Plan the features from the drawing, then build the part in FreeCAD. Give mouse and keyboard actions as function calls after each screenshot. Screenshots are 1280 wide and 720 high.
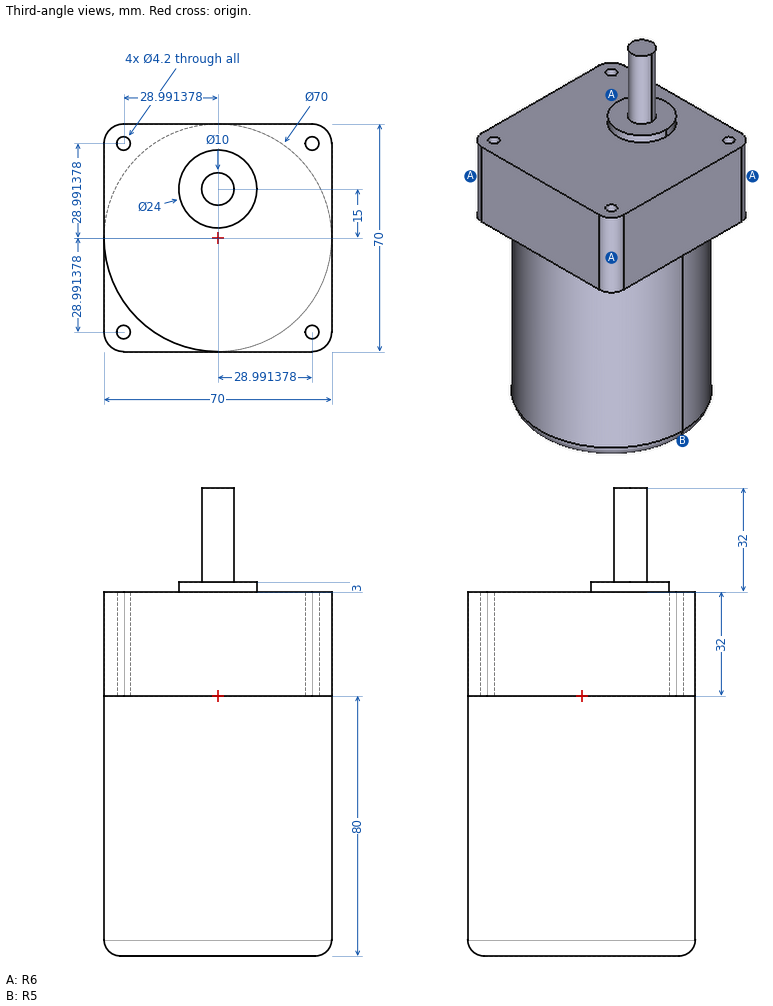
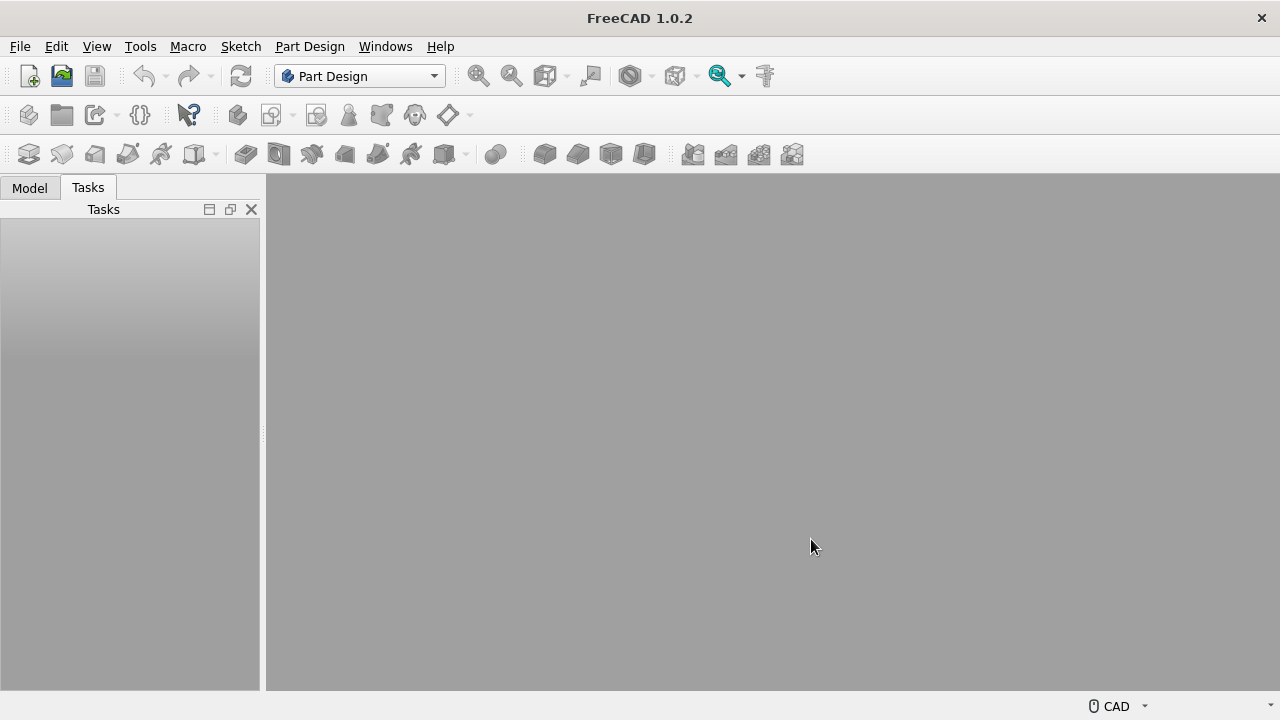
click(29, 76)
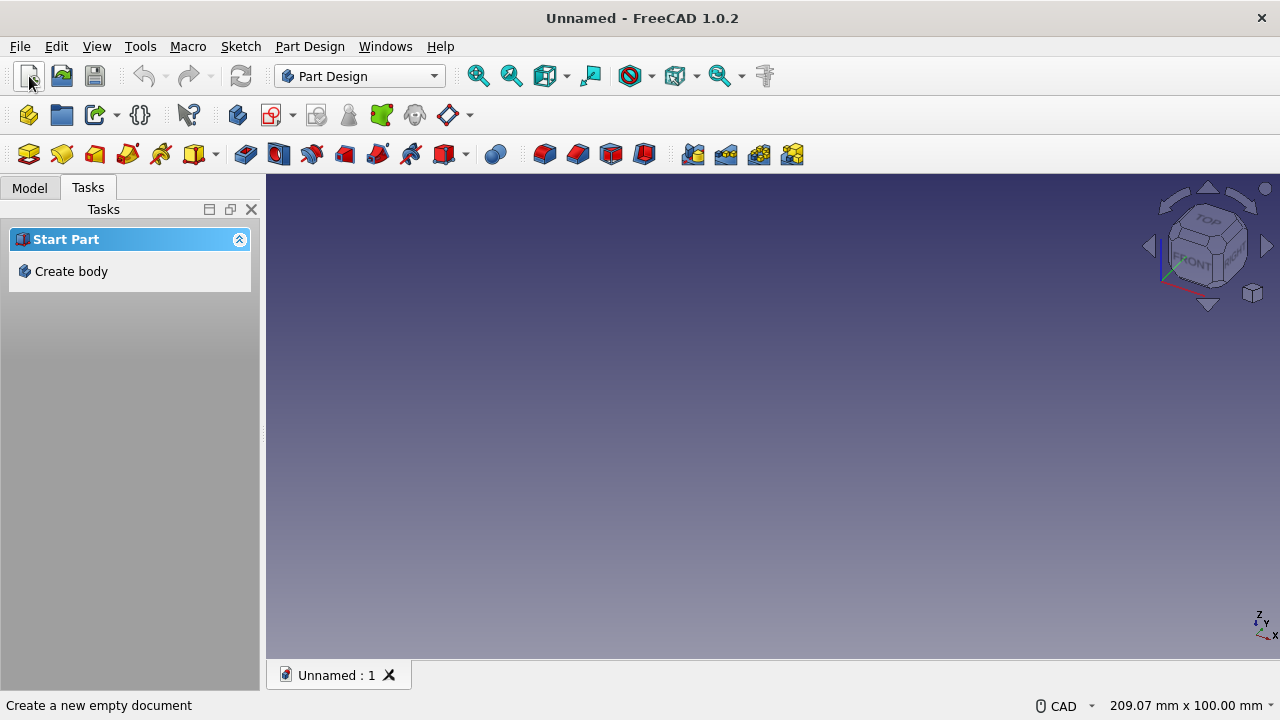
click(270, 116)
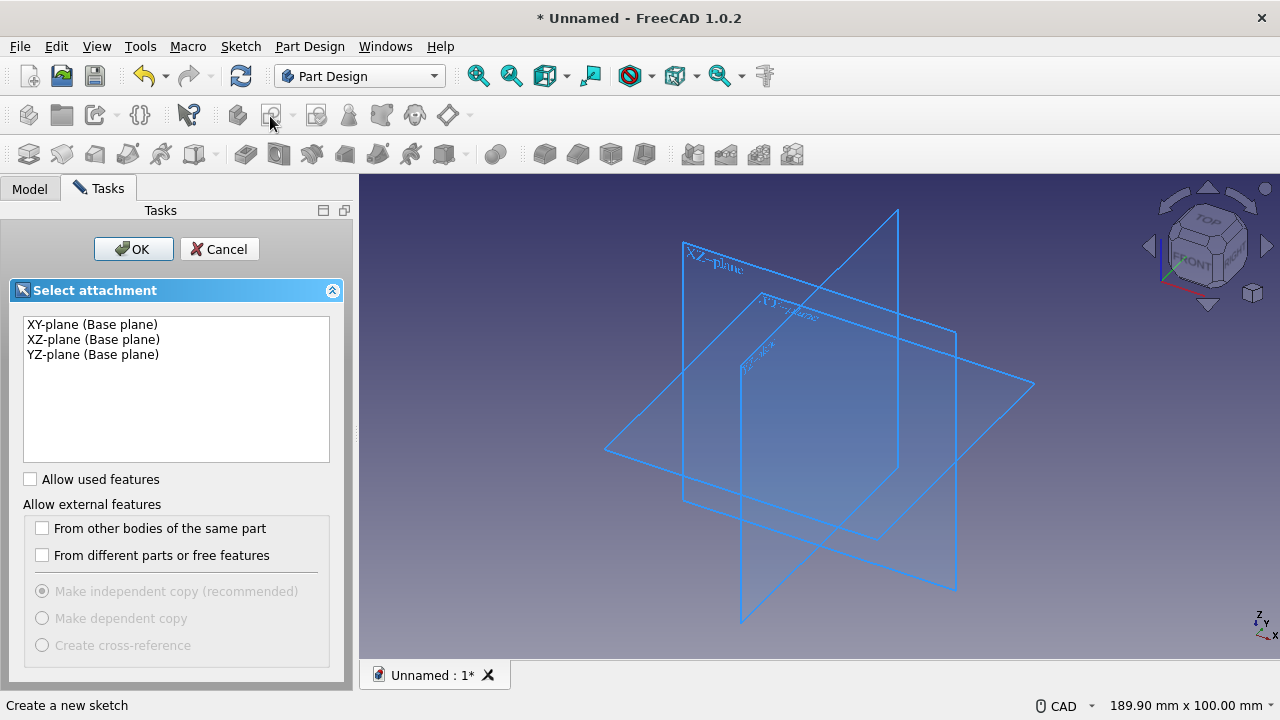
click(84, 324)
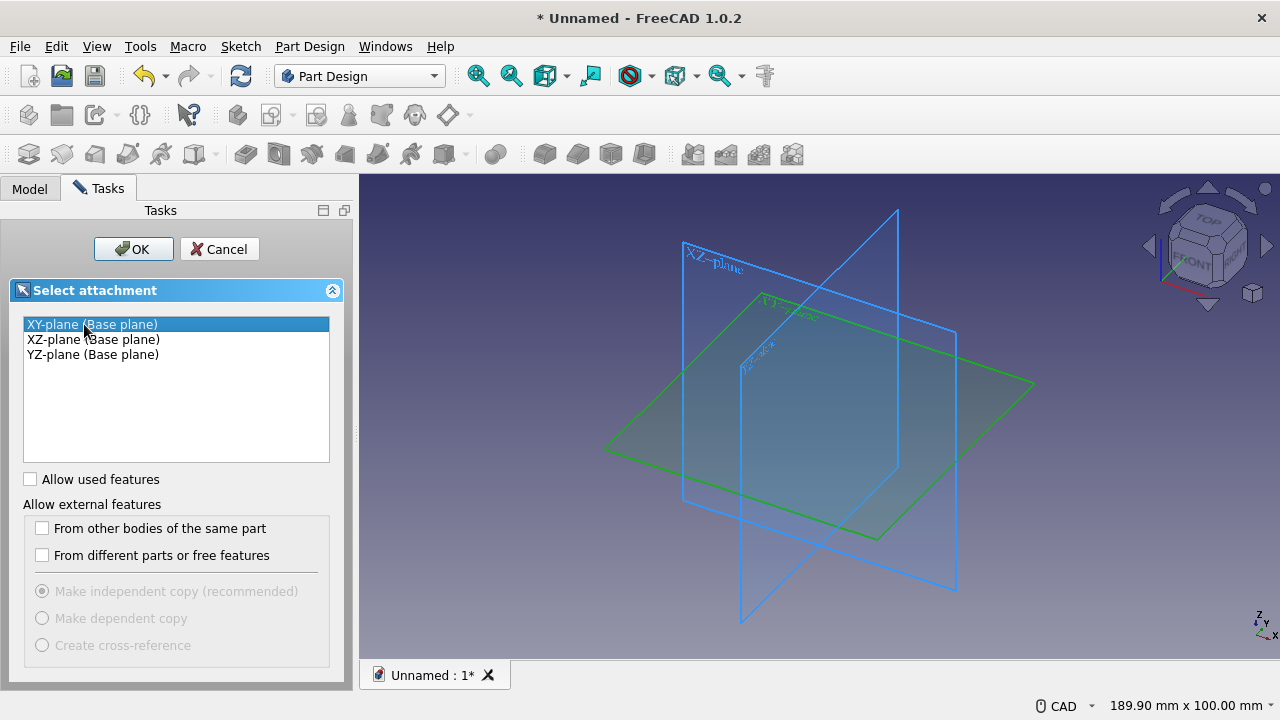
click(134, 249)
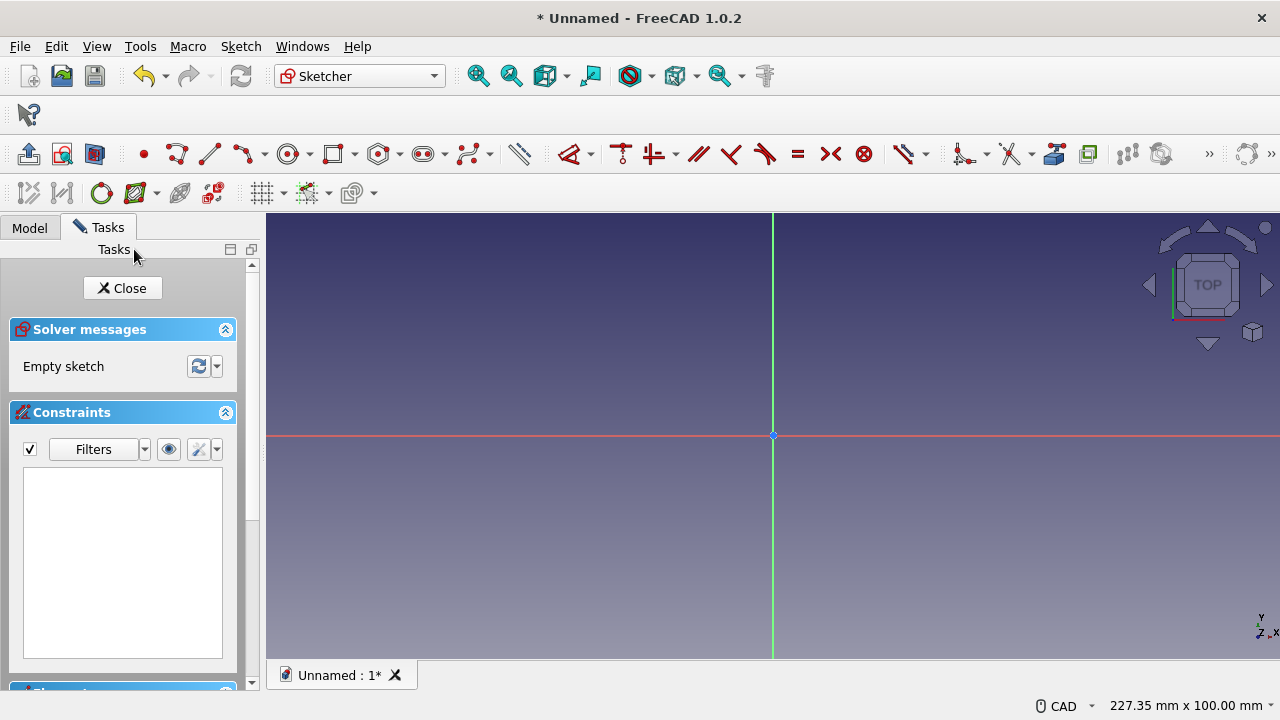
click(354, 154)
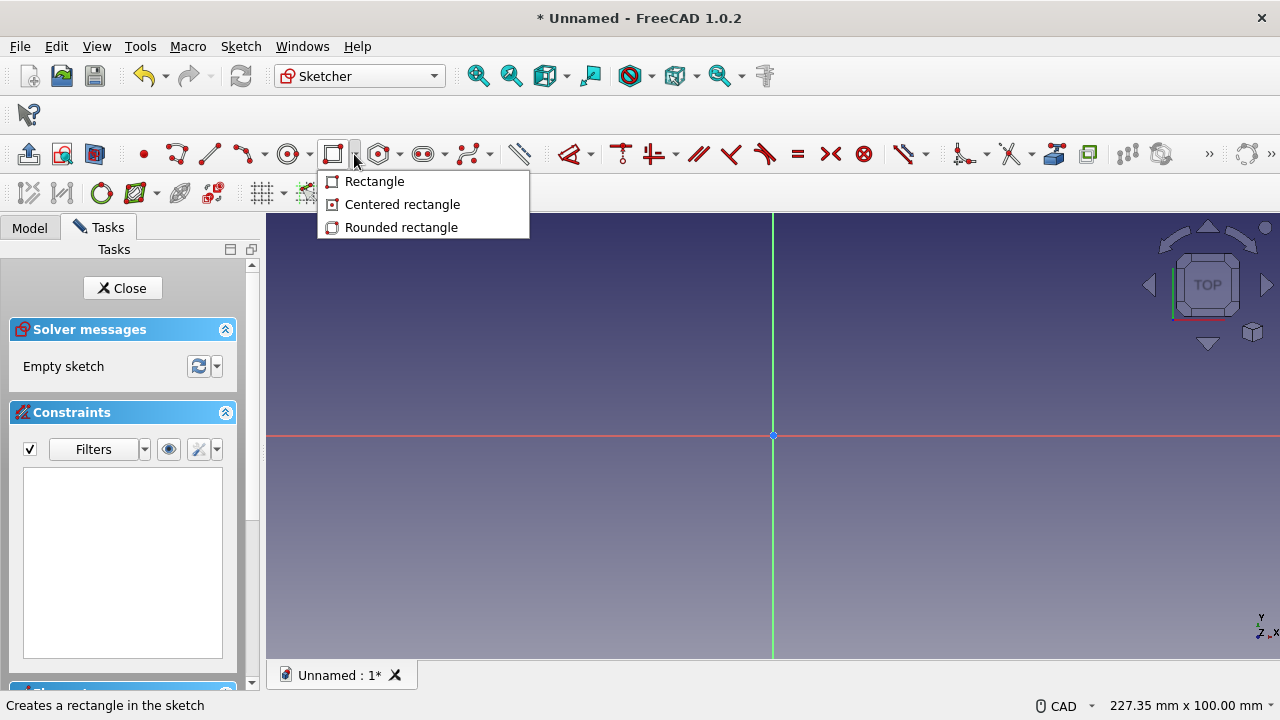
click(424, 204)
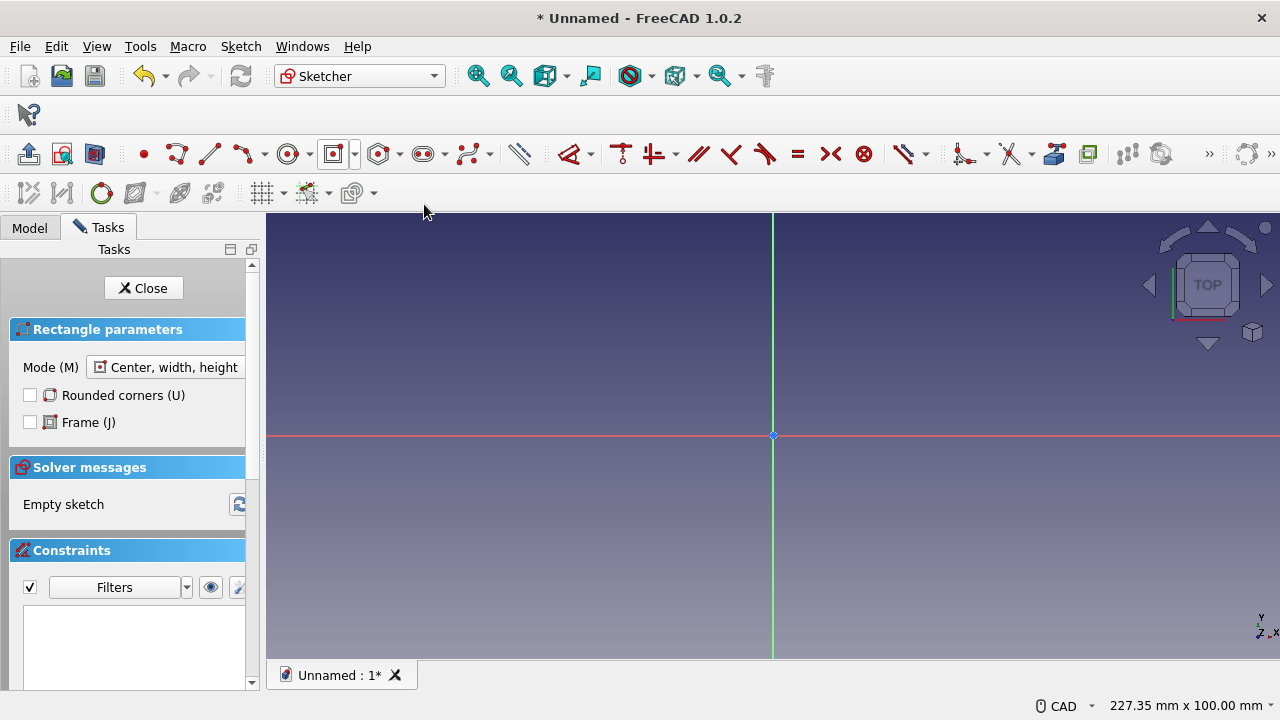
click(773, 436)
move(929, 280)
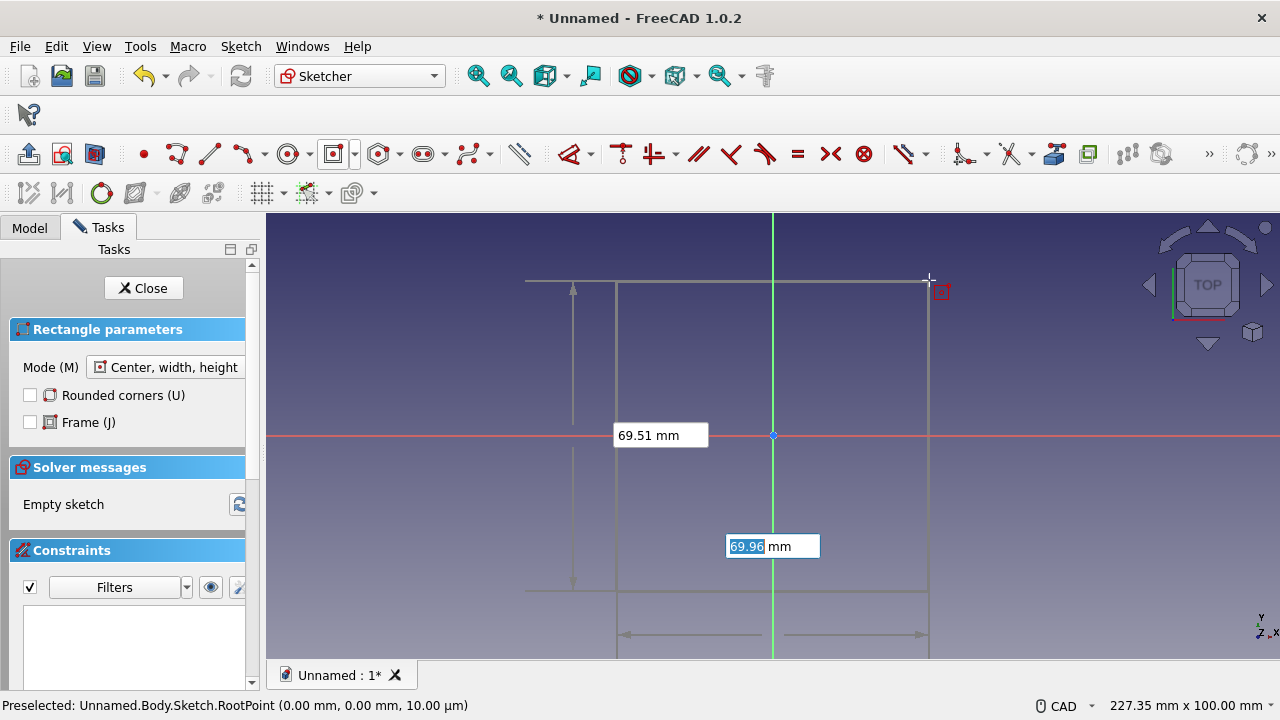
text(70)
key(Tab)
text(70)
key(Return)
key(Escape)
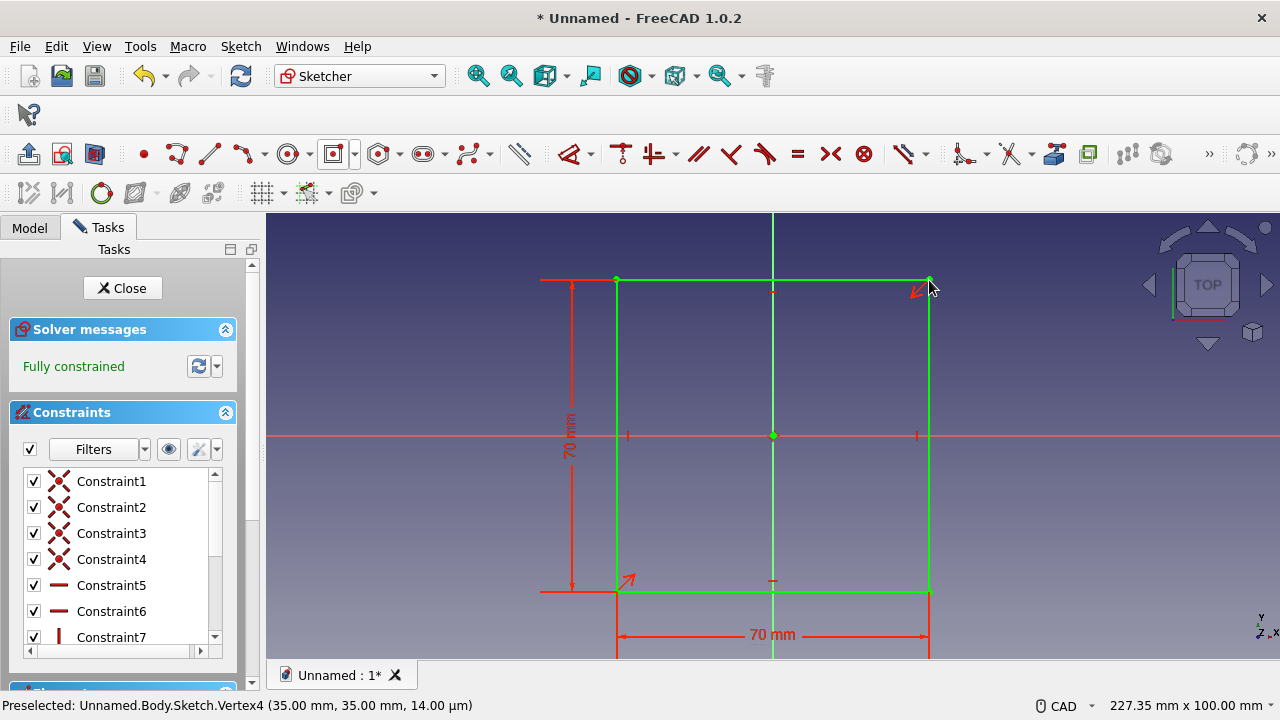
click(123, 288)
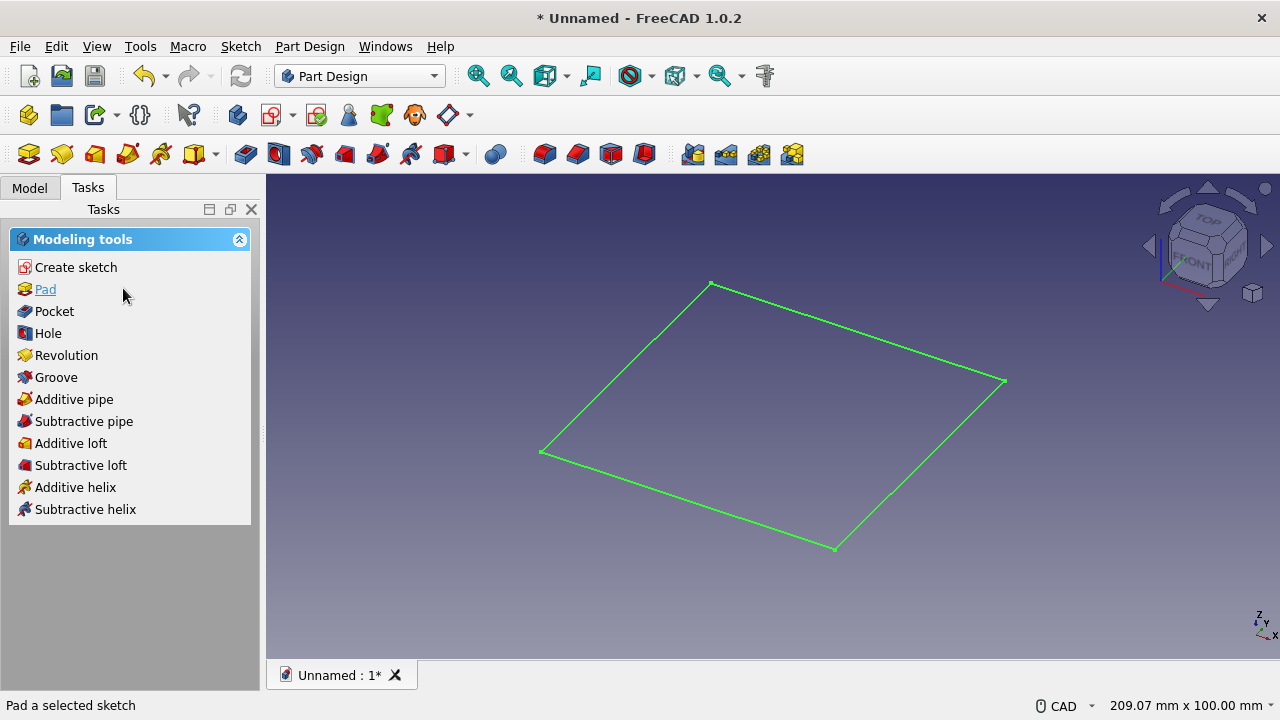
click(29, 154)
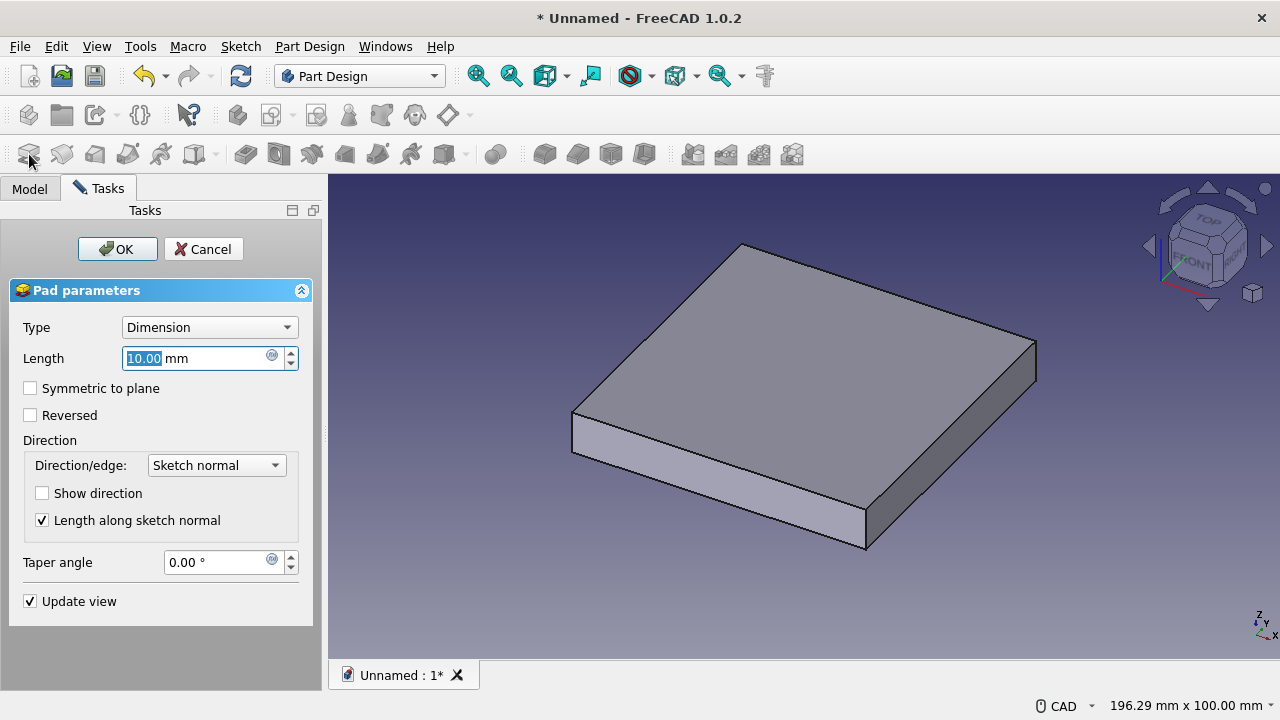
text(32)
key(Tab)